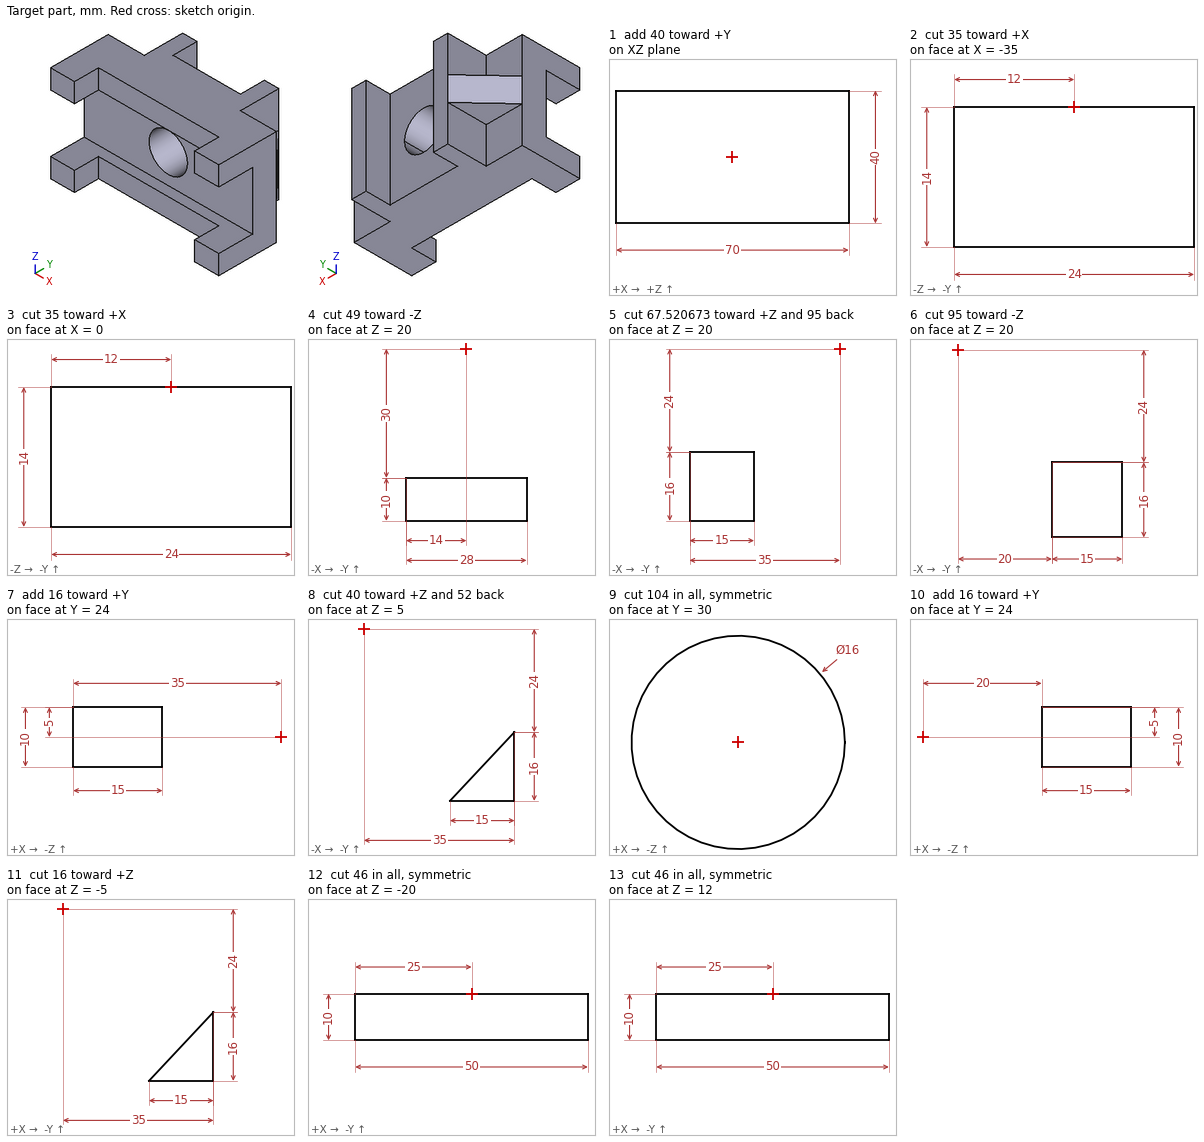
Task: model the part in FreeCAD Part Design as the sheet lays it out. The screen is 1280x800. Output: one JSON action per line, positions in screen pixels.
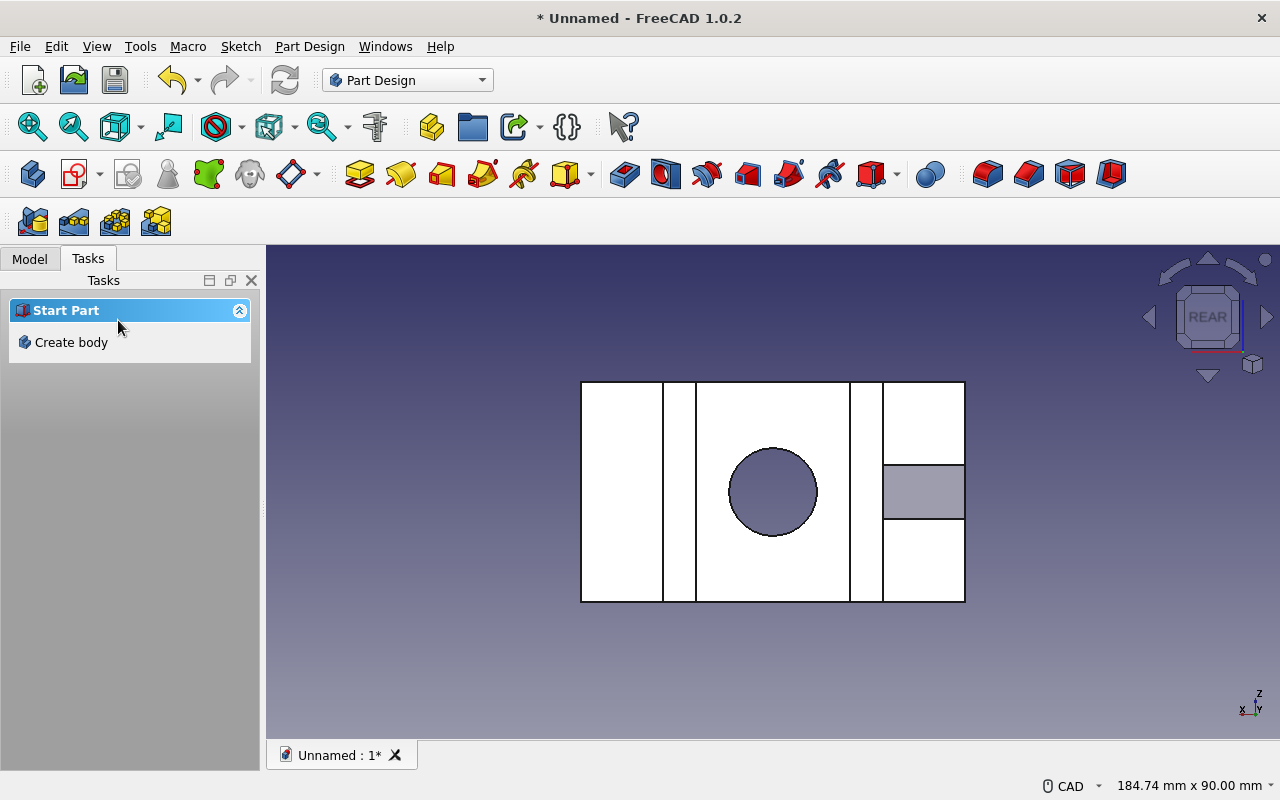
{"action": "key", "text": "v f"}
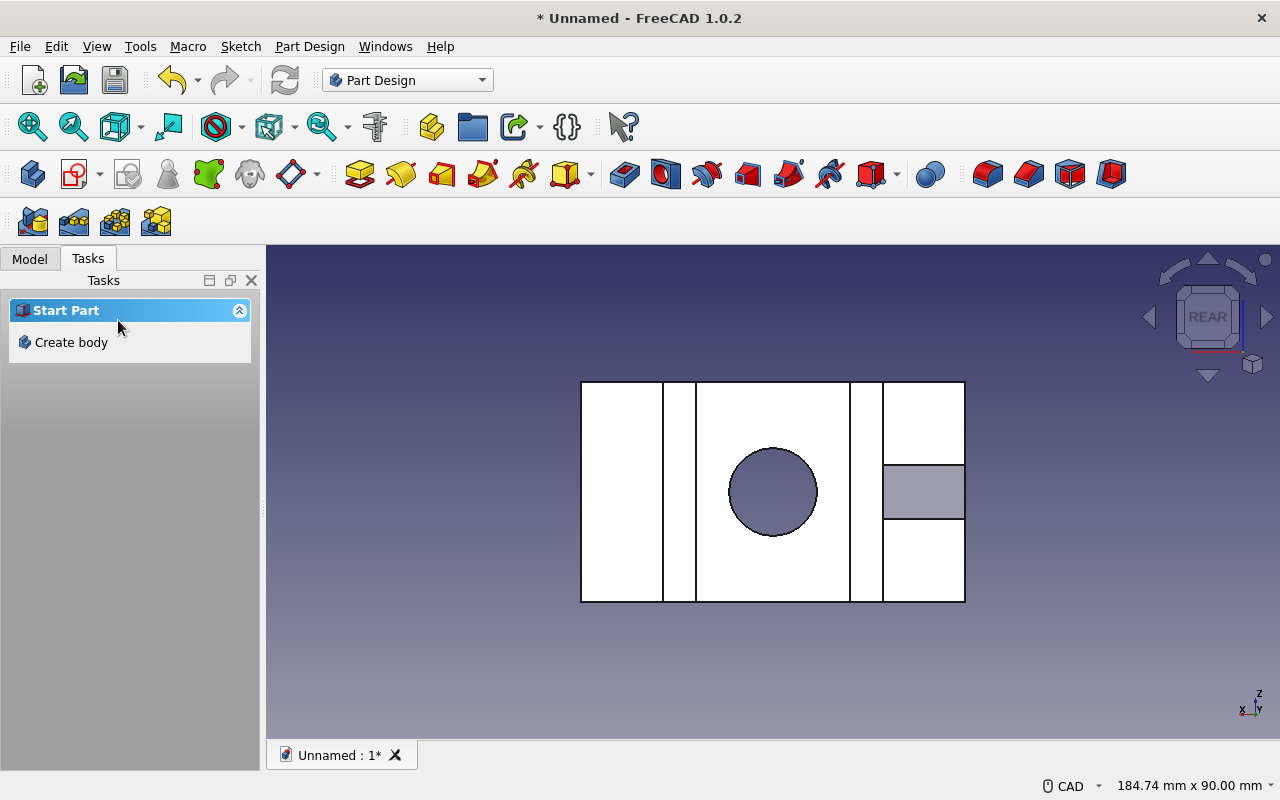
{"action": "left_click", "coordinate": [622, 460]}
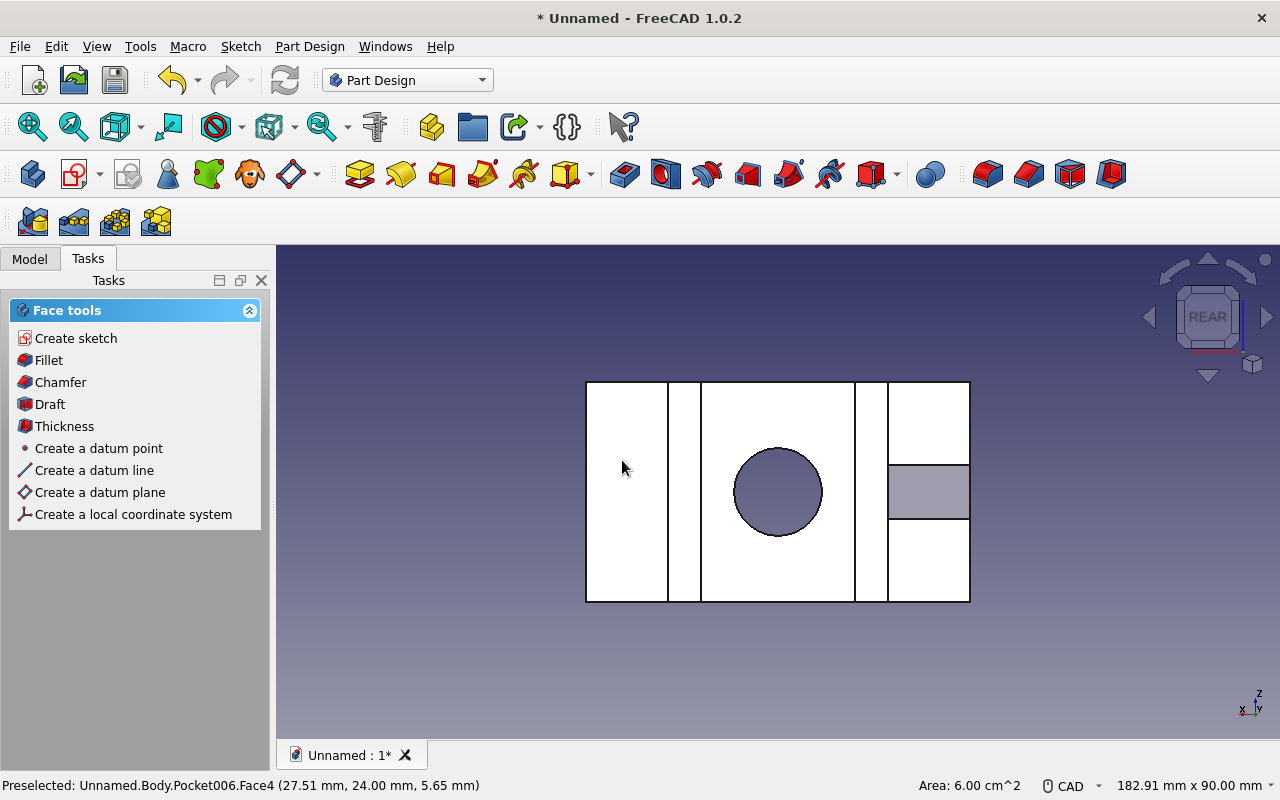
{"action": "left_click", "coordinate": [74, 174]}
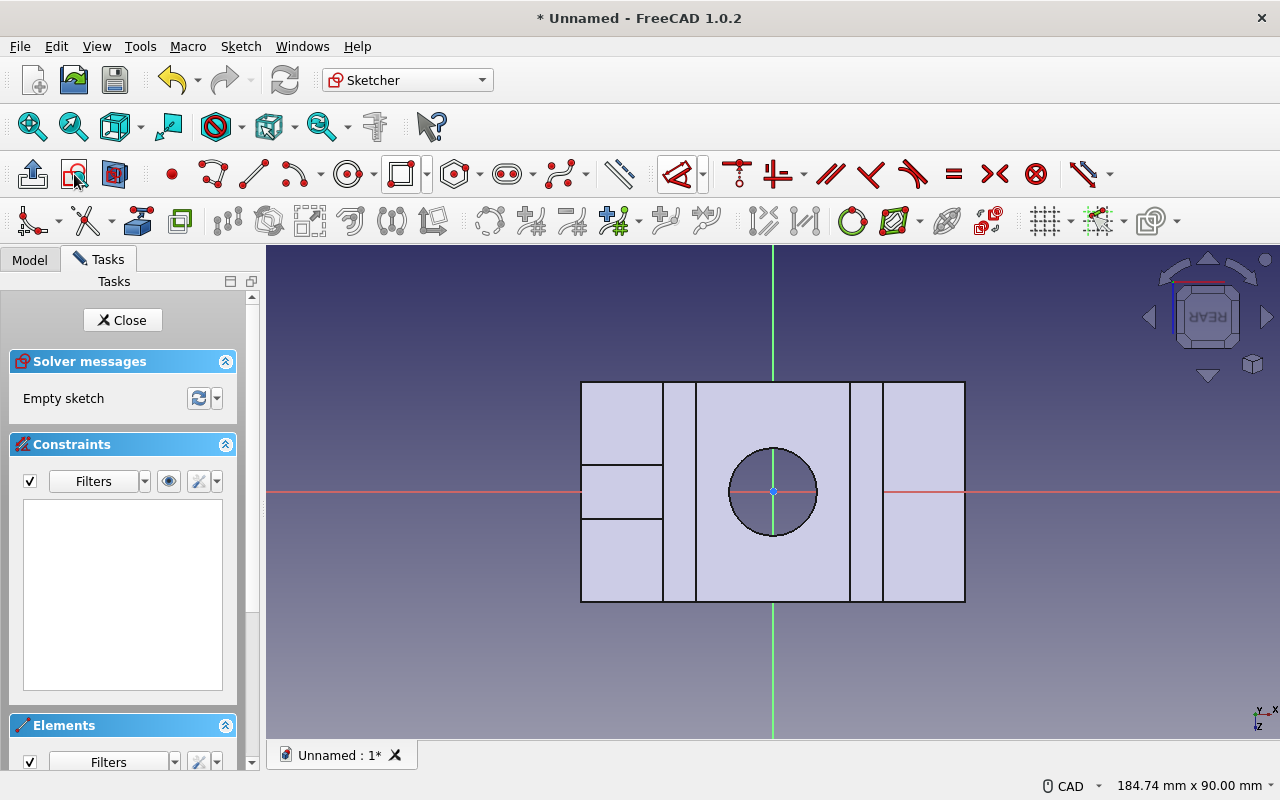
{"action": "scroll", "coordinate": [940, 492], "scroll_direction": "up", "scroll_amount": 6}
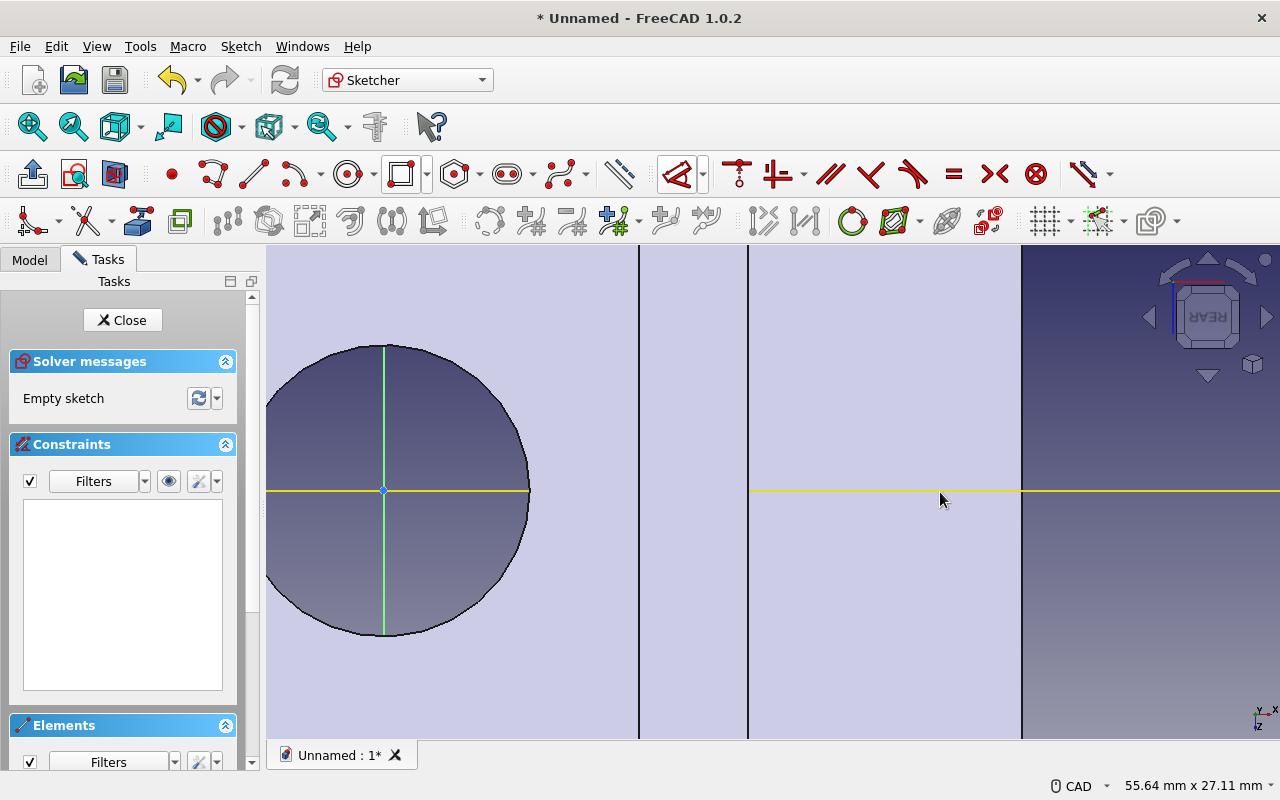
{"action": "left_click", "coordinate": [400, 174]}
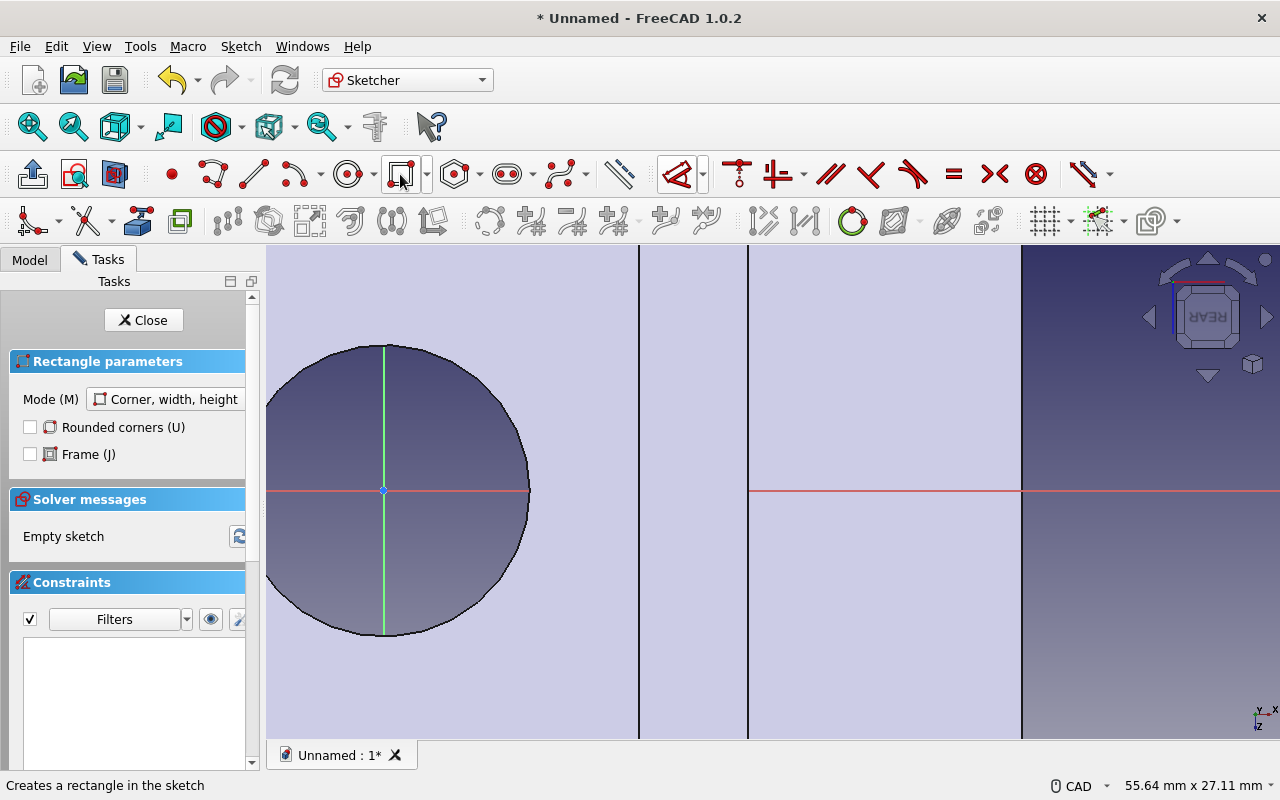
{"action": "left_click", "coordinate": [748, 400]}
{"action": "left_click", "coordinate": [1022, 582]}
{"action": "key", "text": "Escape"}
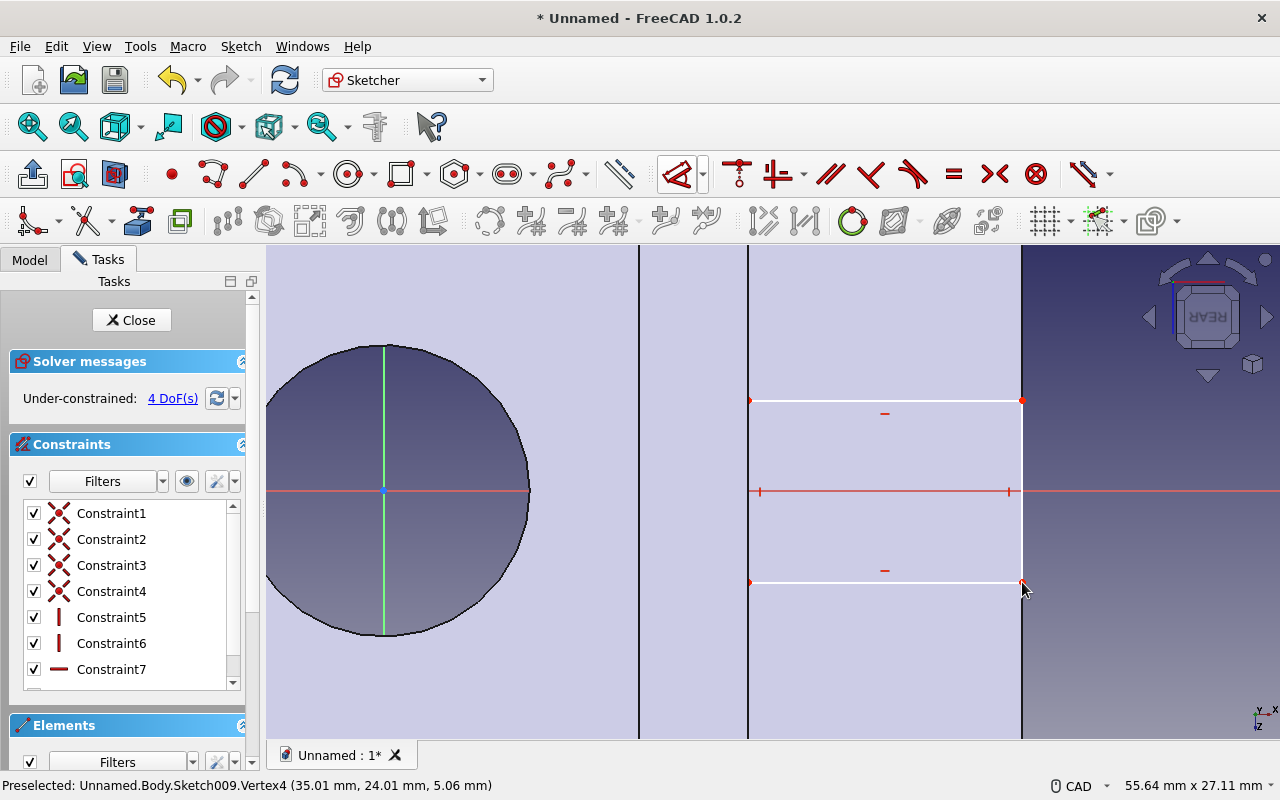
{"action": "left_click", "coordinate": [748, 456]}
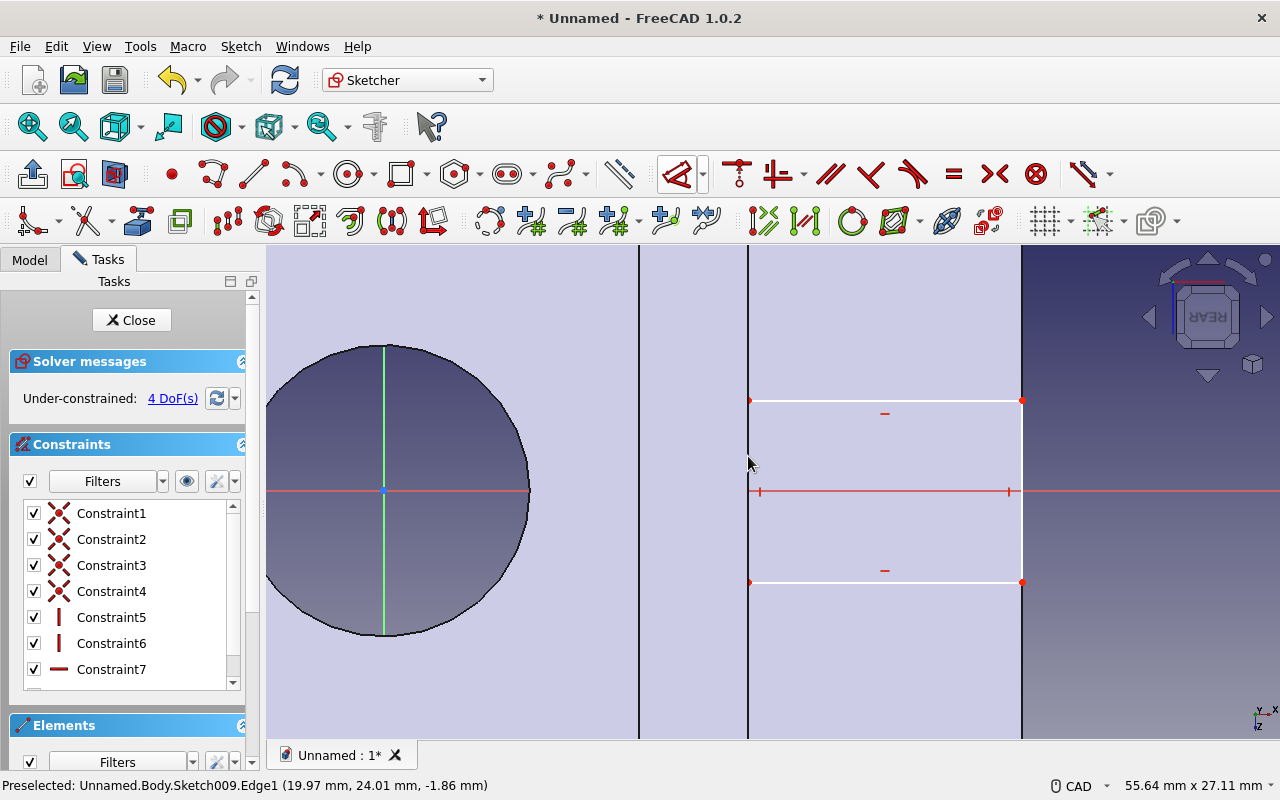
{"action": "key", "text": "i"}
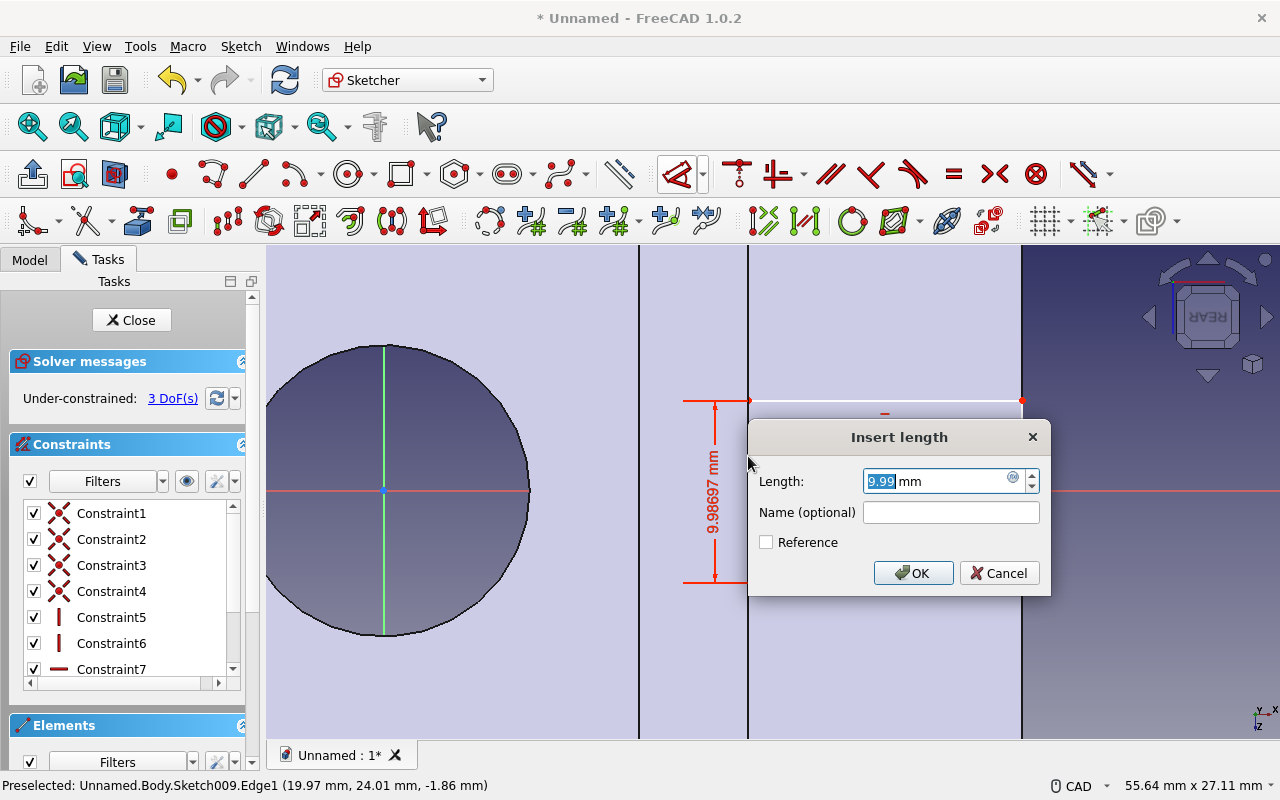
{"action": "type", "text": "10"}
{"action": "key", "text": "Return"}